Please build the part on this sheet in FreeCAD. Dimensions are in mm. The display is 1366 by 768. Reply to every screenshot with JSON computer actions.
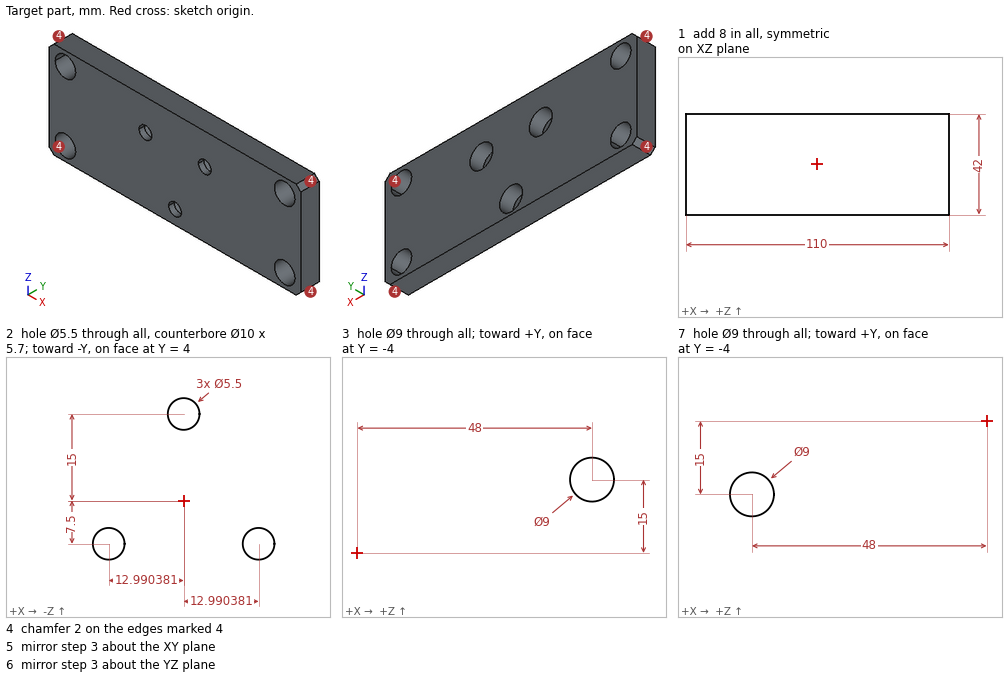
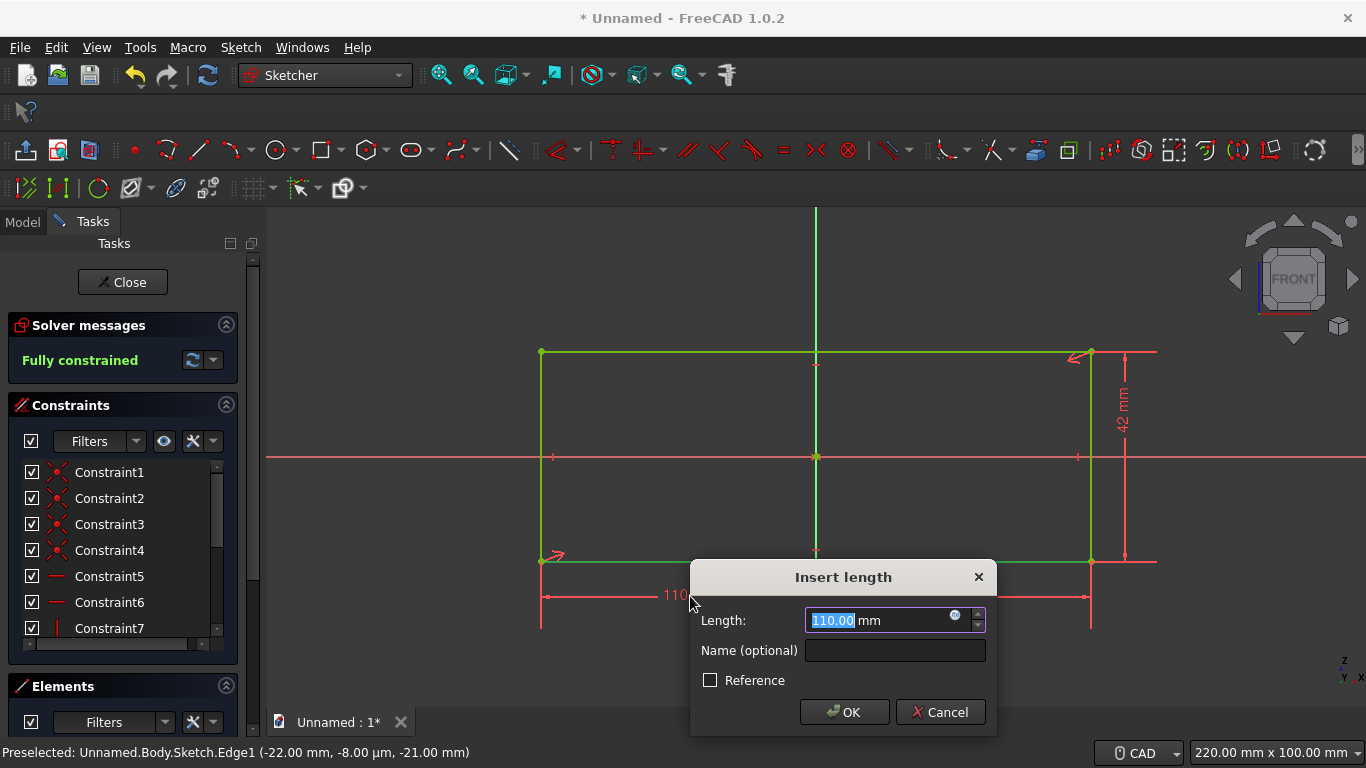
{"action": "type", "text": "110"}
{"action": "key", "text": "Return"}
{"action": "key", "text": "Escape"}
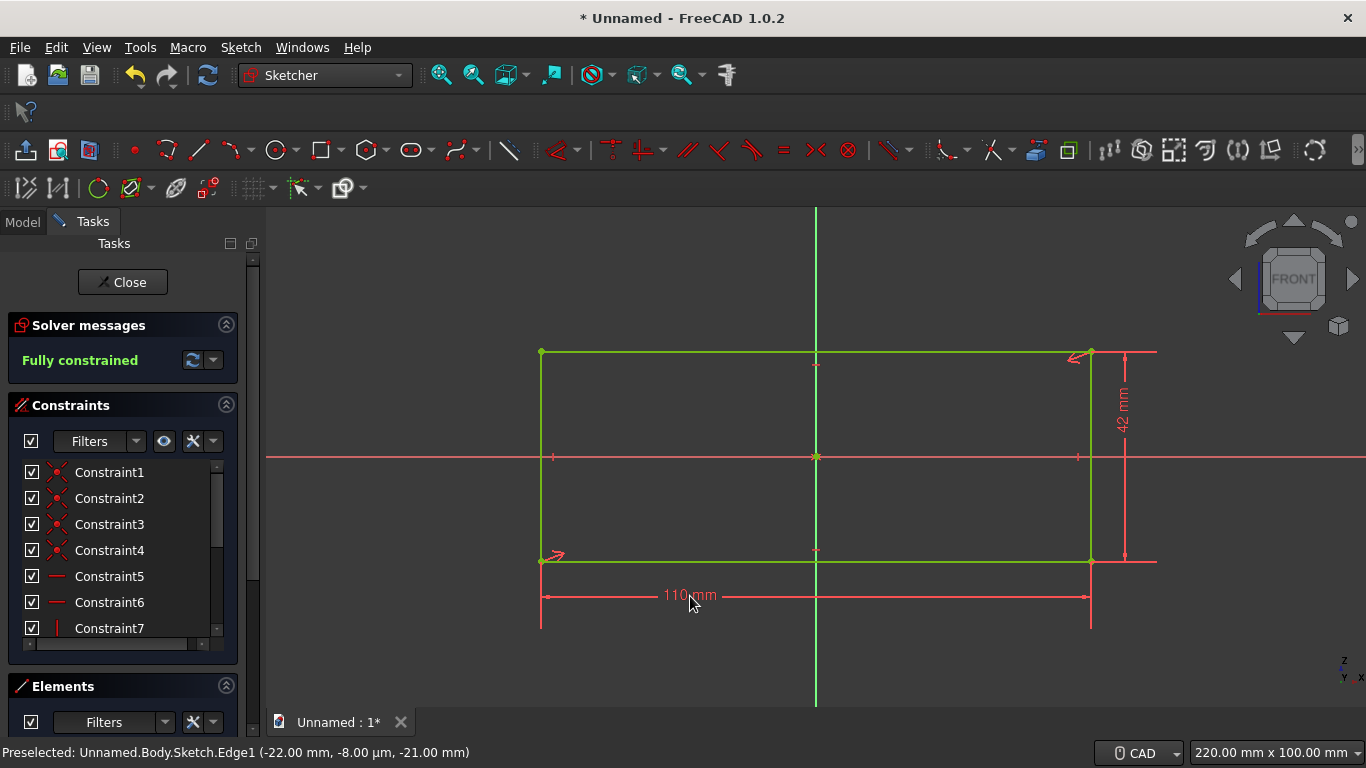
{"action": "left_click", "coordinate": [123, 282]}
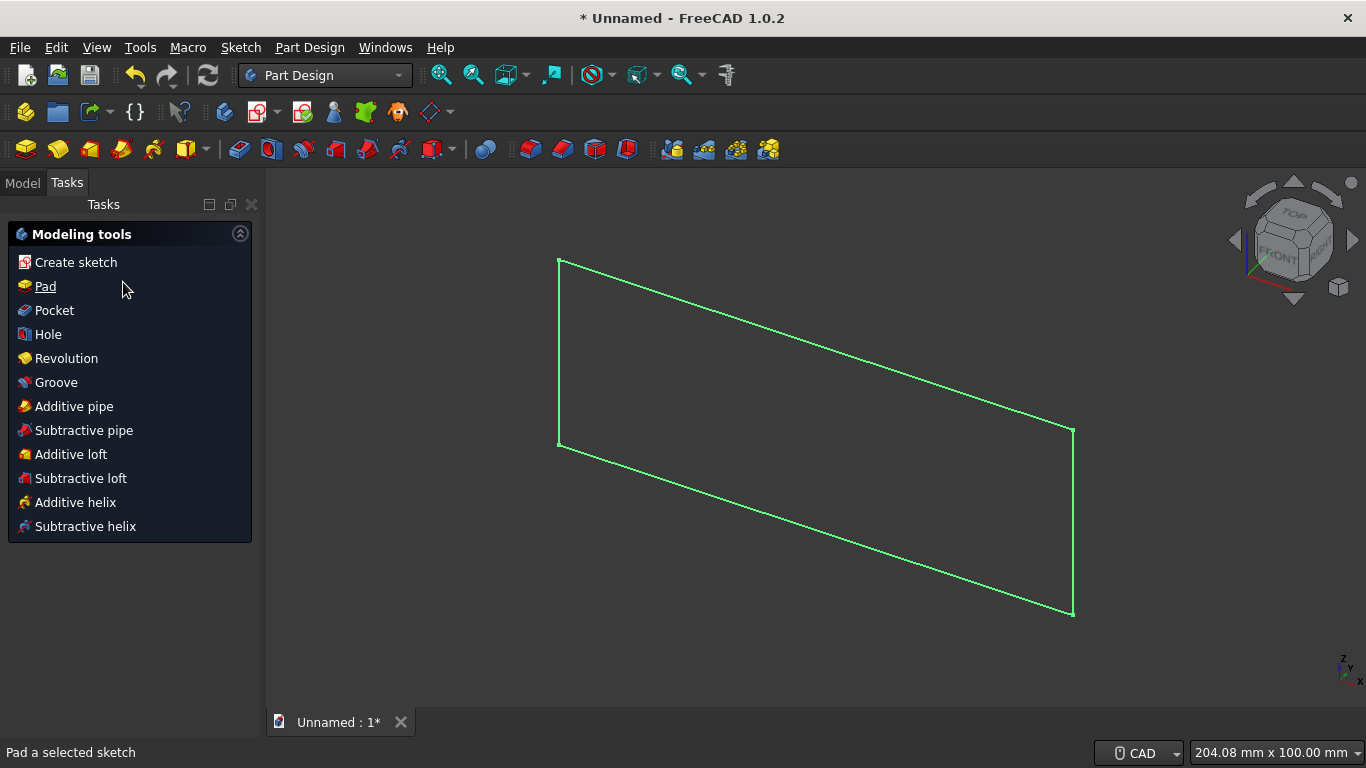
{"action": "left_click", "coordinate": [26, 150]}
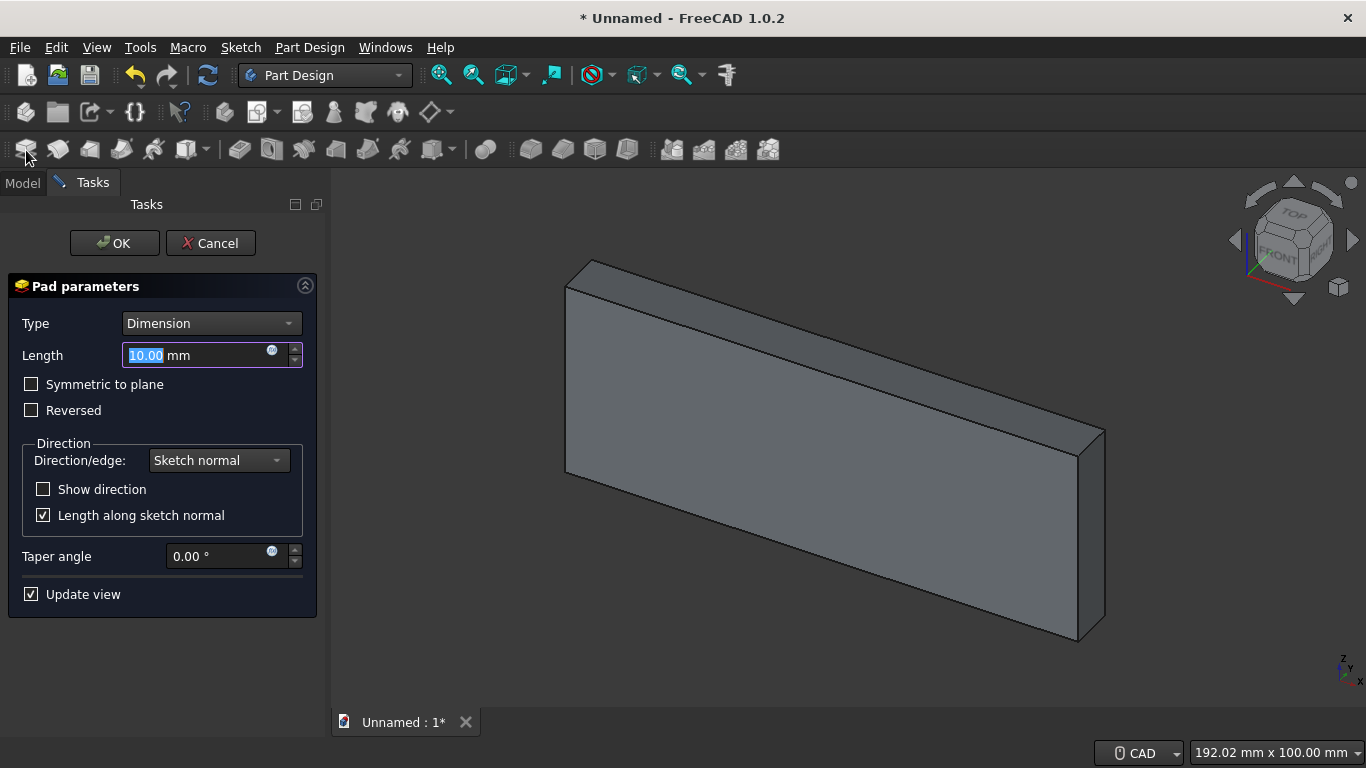
{"action": "type", "text": "8"}
{"action": "key", "text": "Tab"}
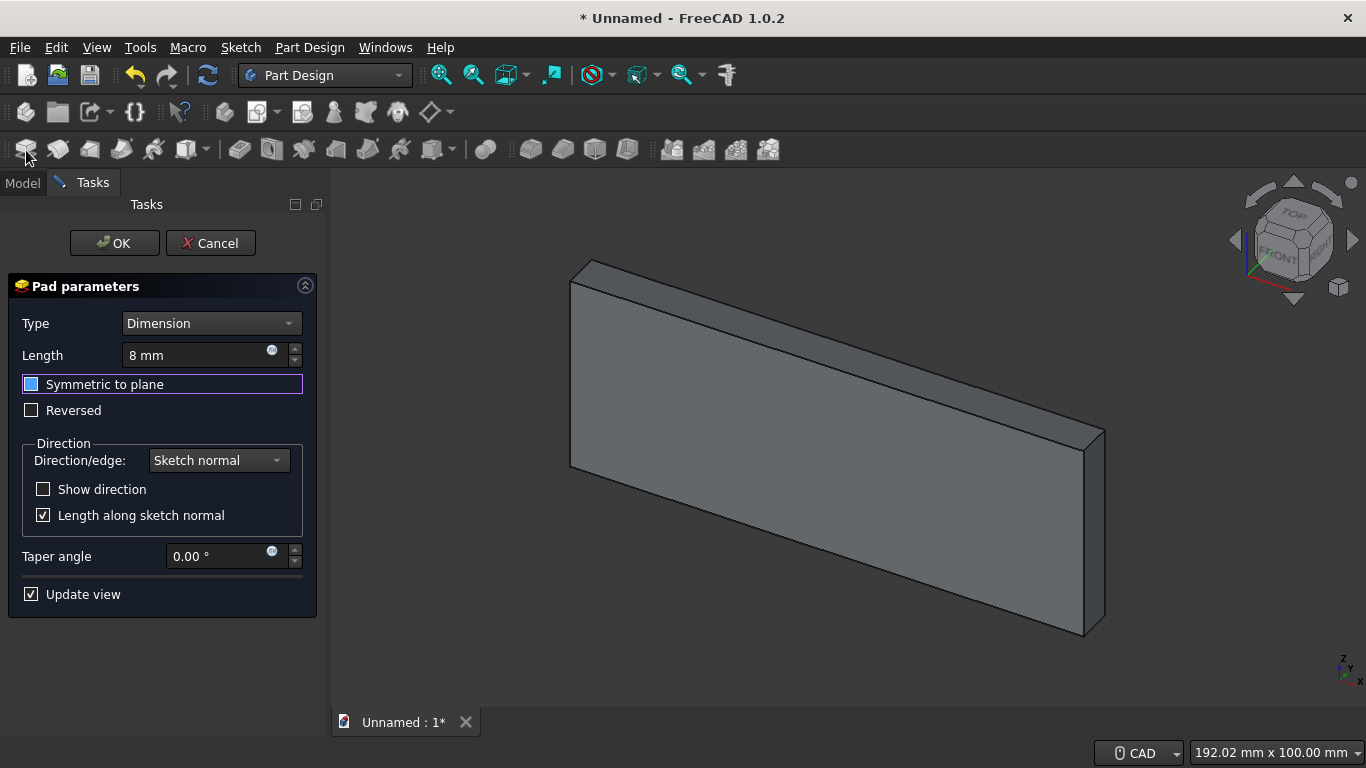
{"action": "left_click", "coordinate": [30, 384]}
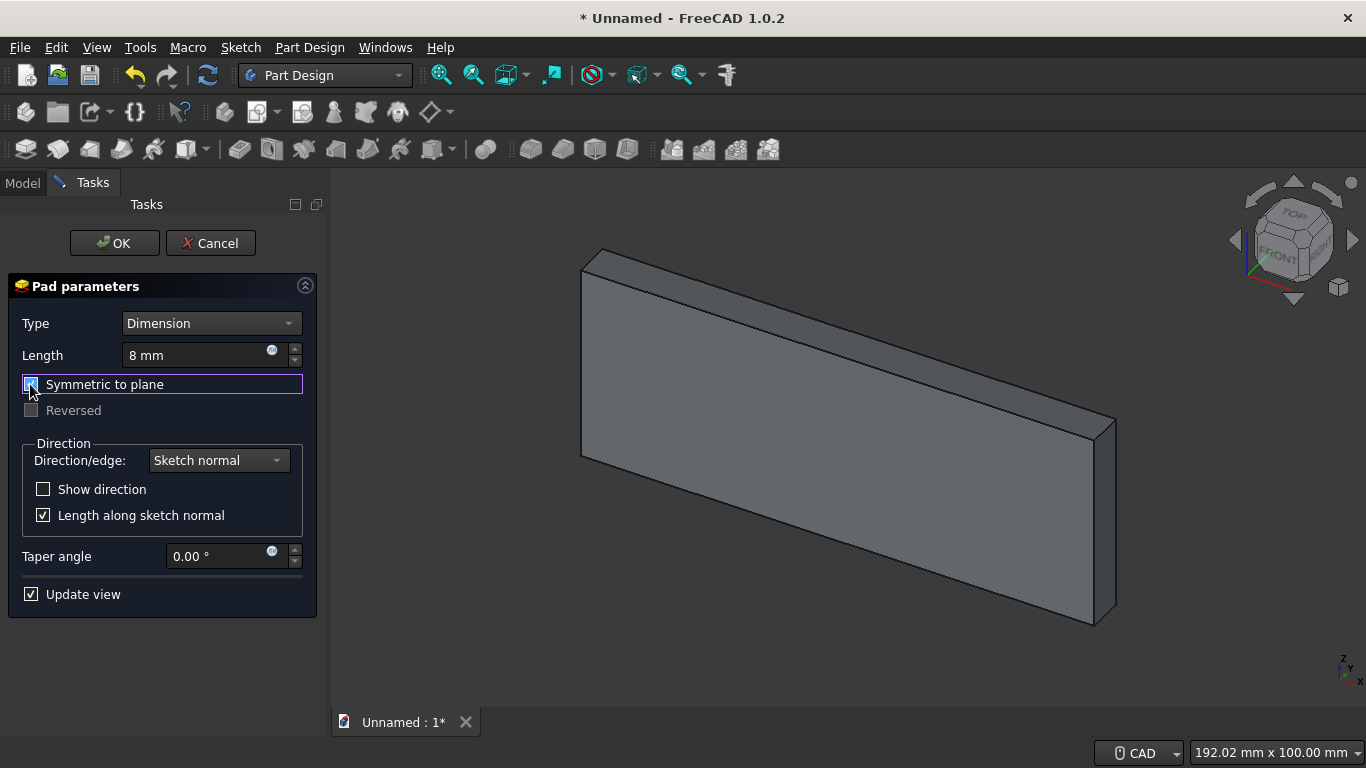
{"action": "left_click", "coordinate": [115, 243]}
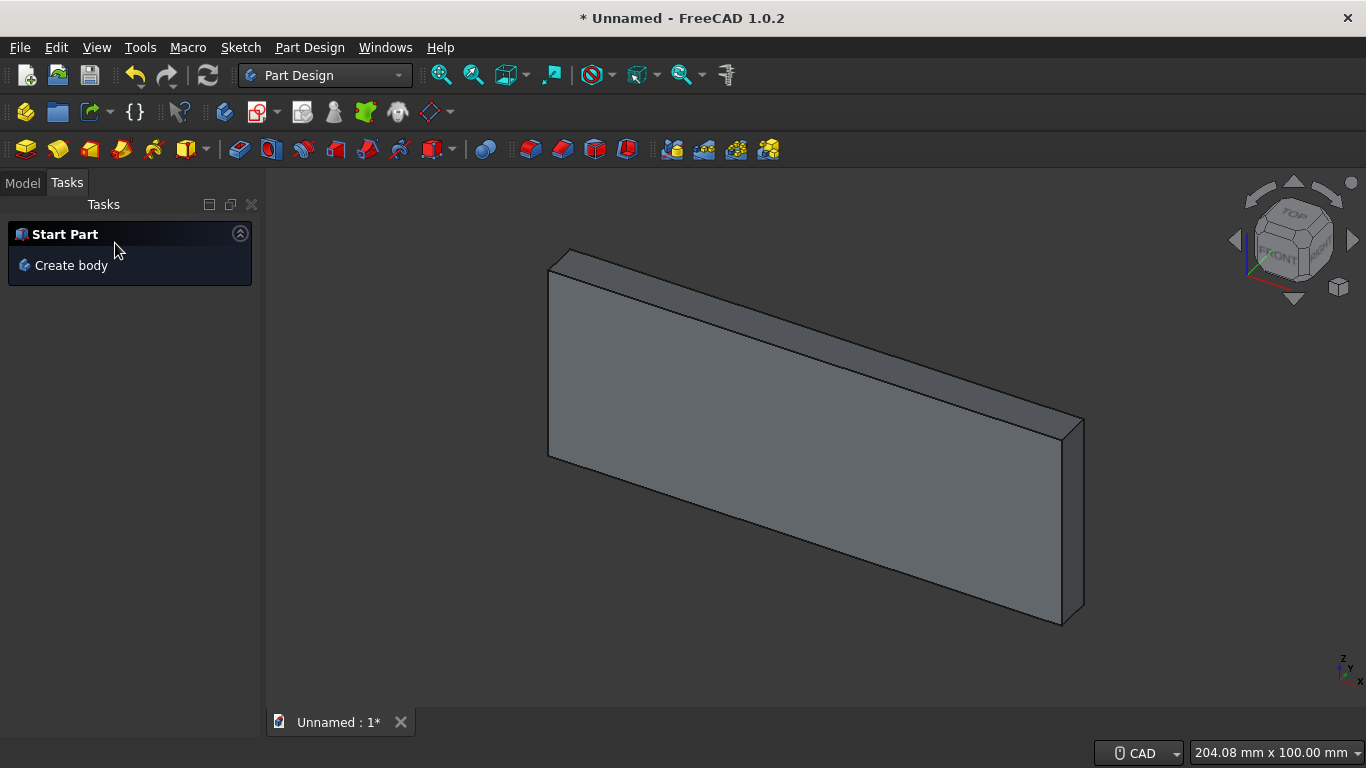
{"action": "key", "text": "4"}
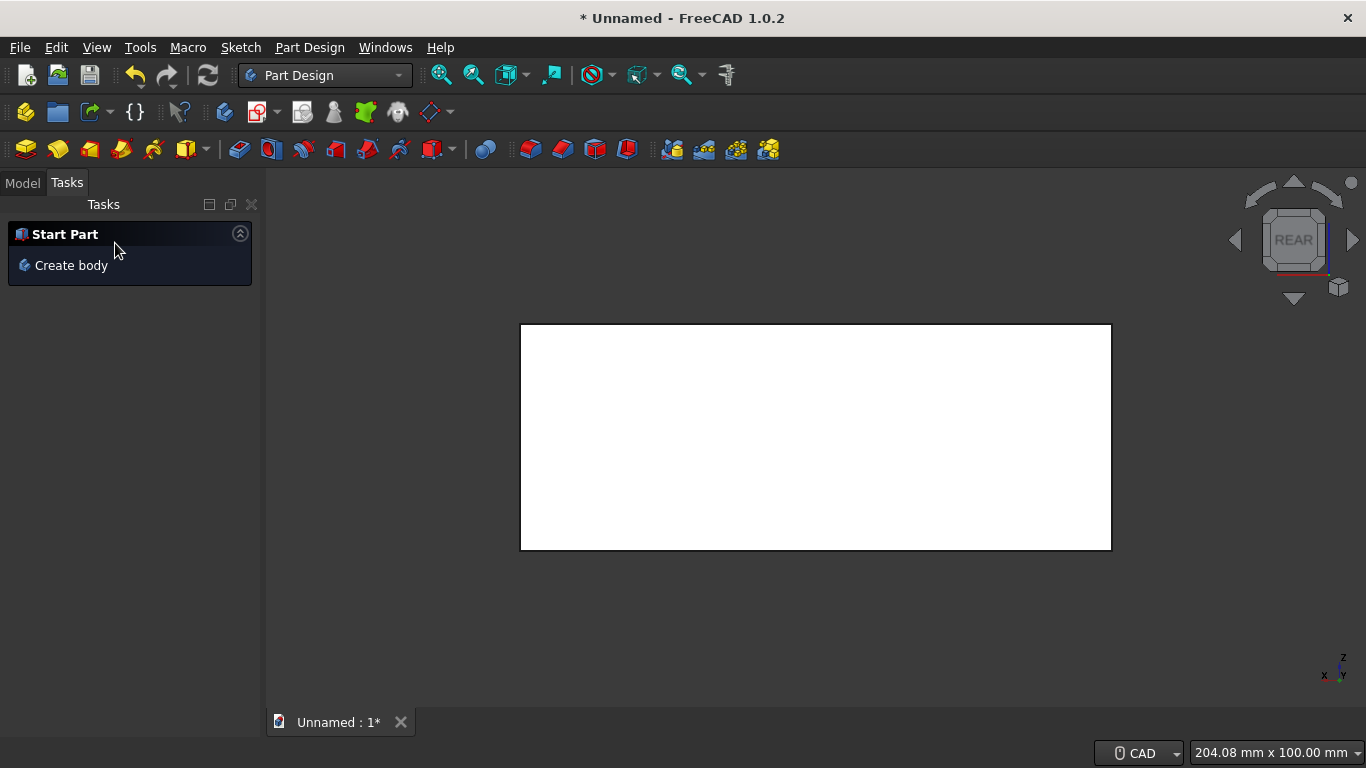
{"action": "left_click", "coordinate": [647, 436]}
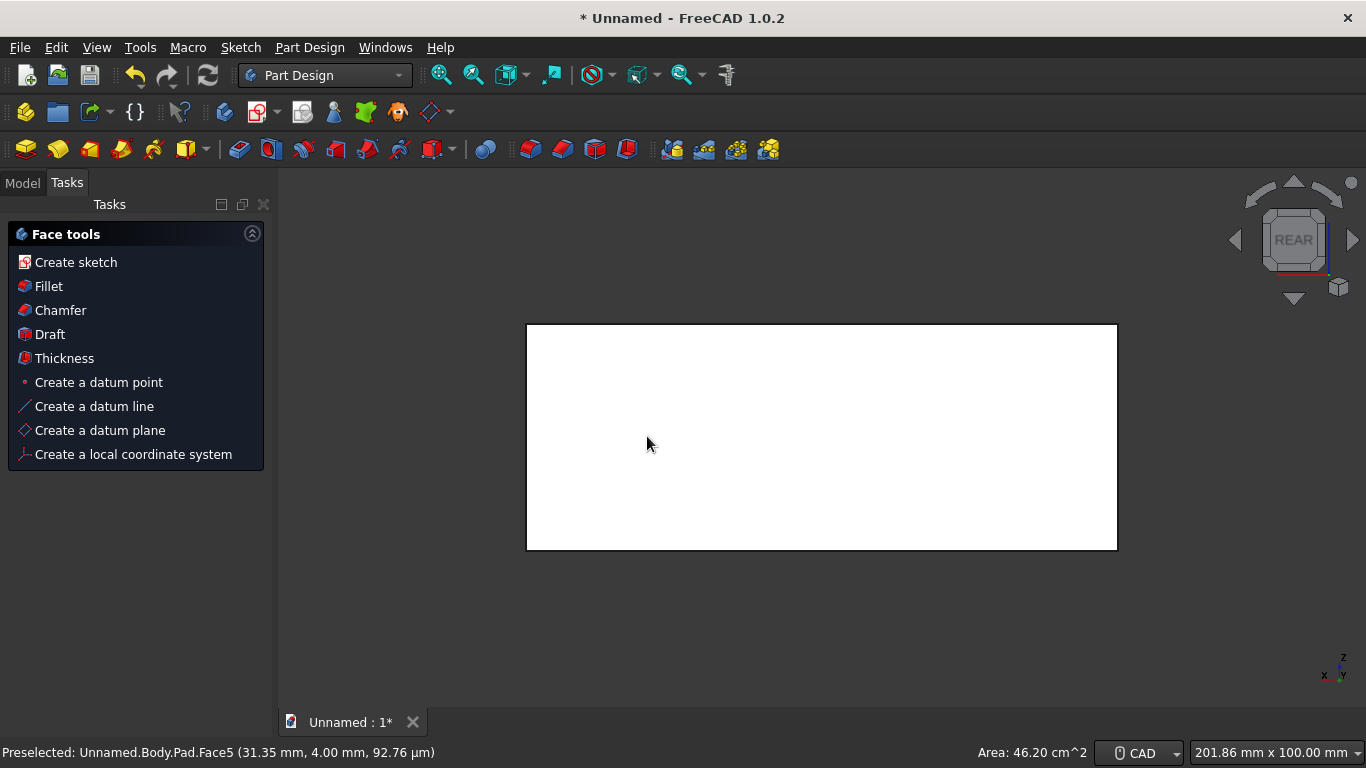
{"action": "left_click", "coordinate": [258, 112]}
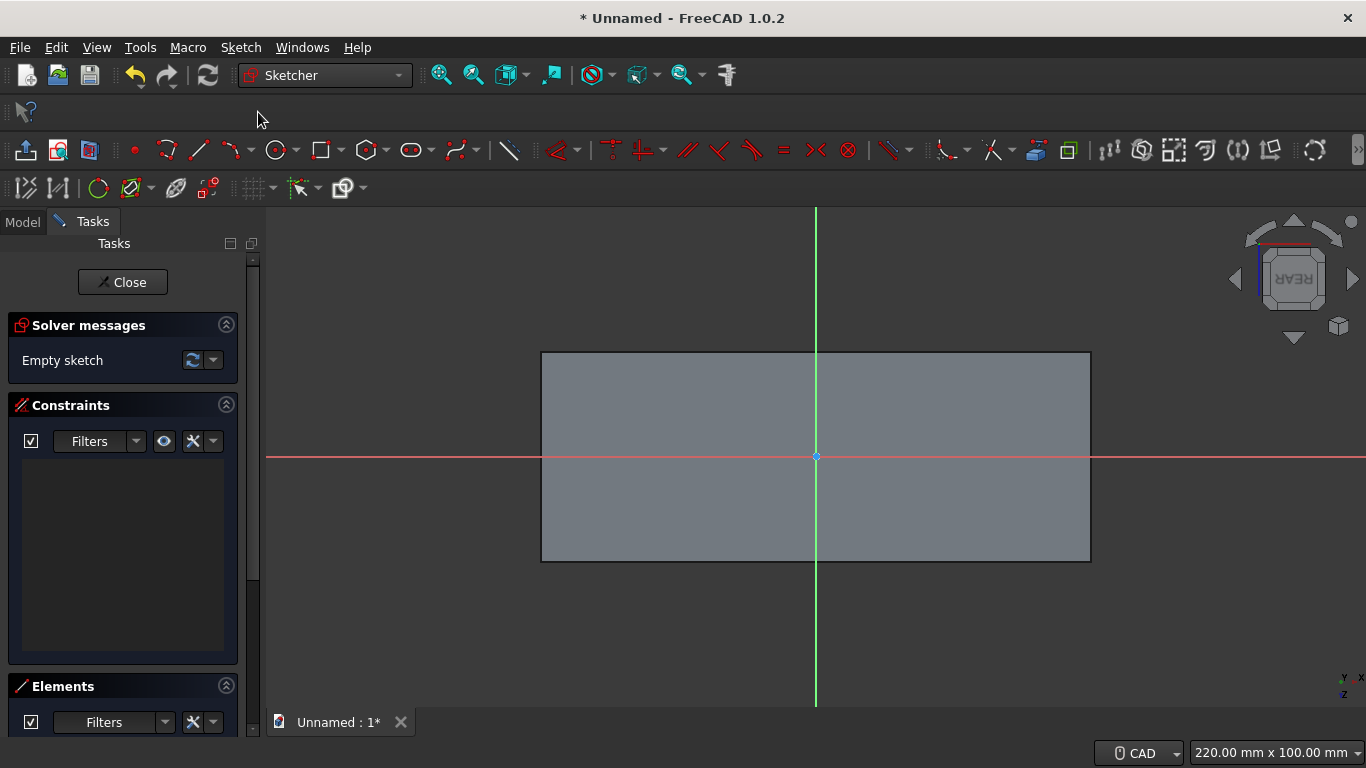
{"action": "scroll", "coordinate": [872, 423], "scroll_direction": "up", "scroll_amount": 4}